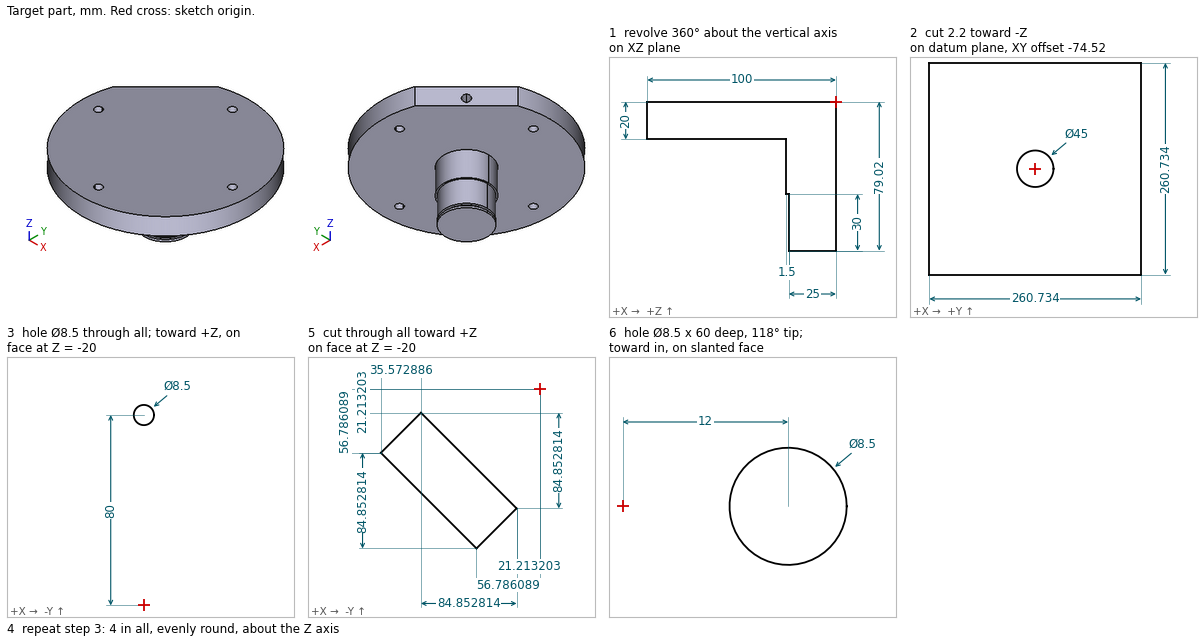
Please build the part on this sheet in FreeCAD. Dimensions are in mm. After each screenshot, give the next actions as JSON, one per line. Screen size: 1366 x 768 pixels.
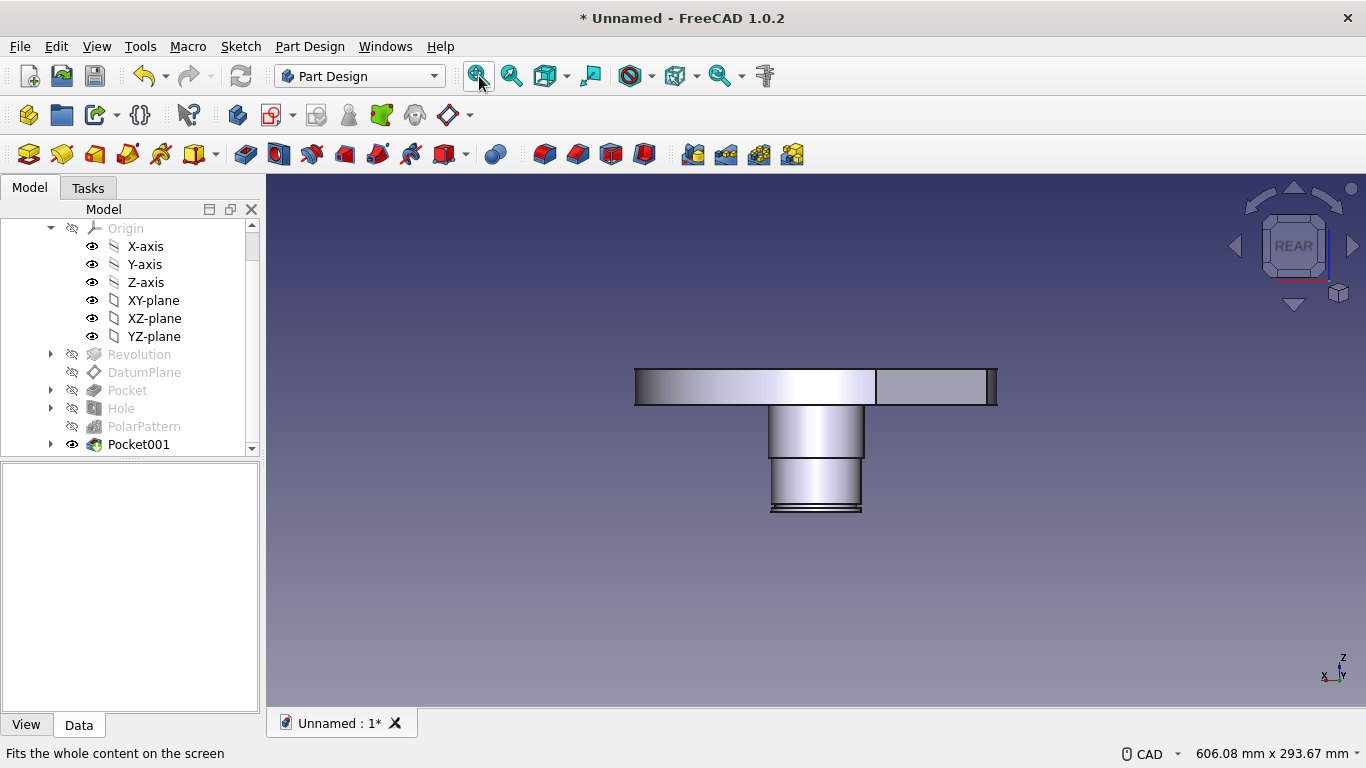
{"action": "left_click", "coordinate": [963, 386]}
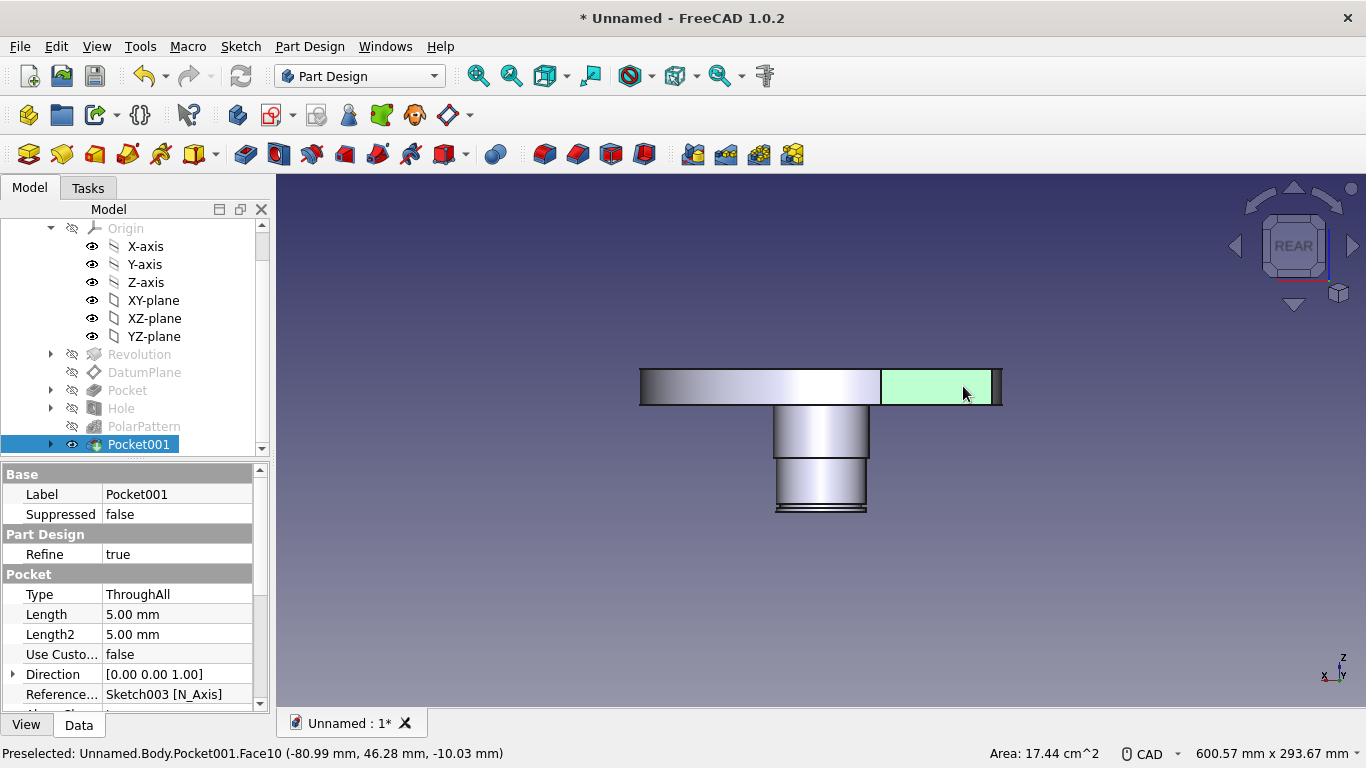
{"action": "left_click", "coordinate": [270, 116]}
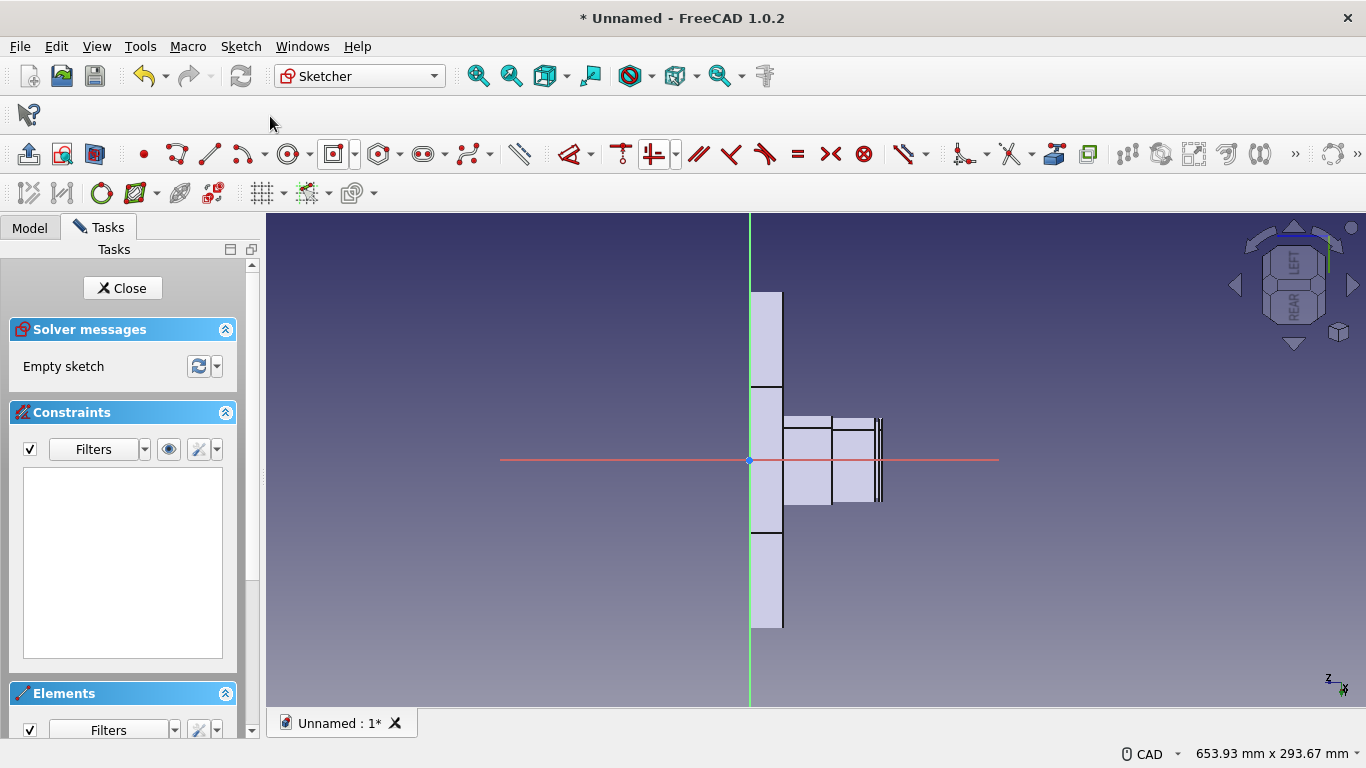
{"action": "left_click", "coordinate": [95, 154]}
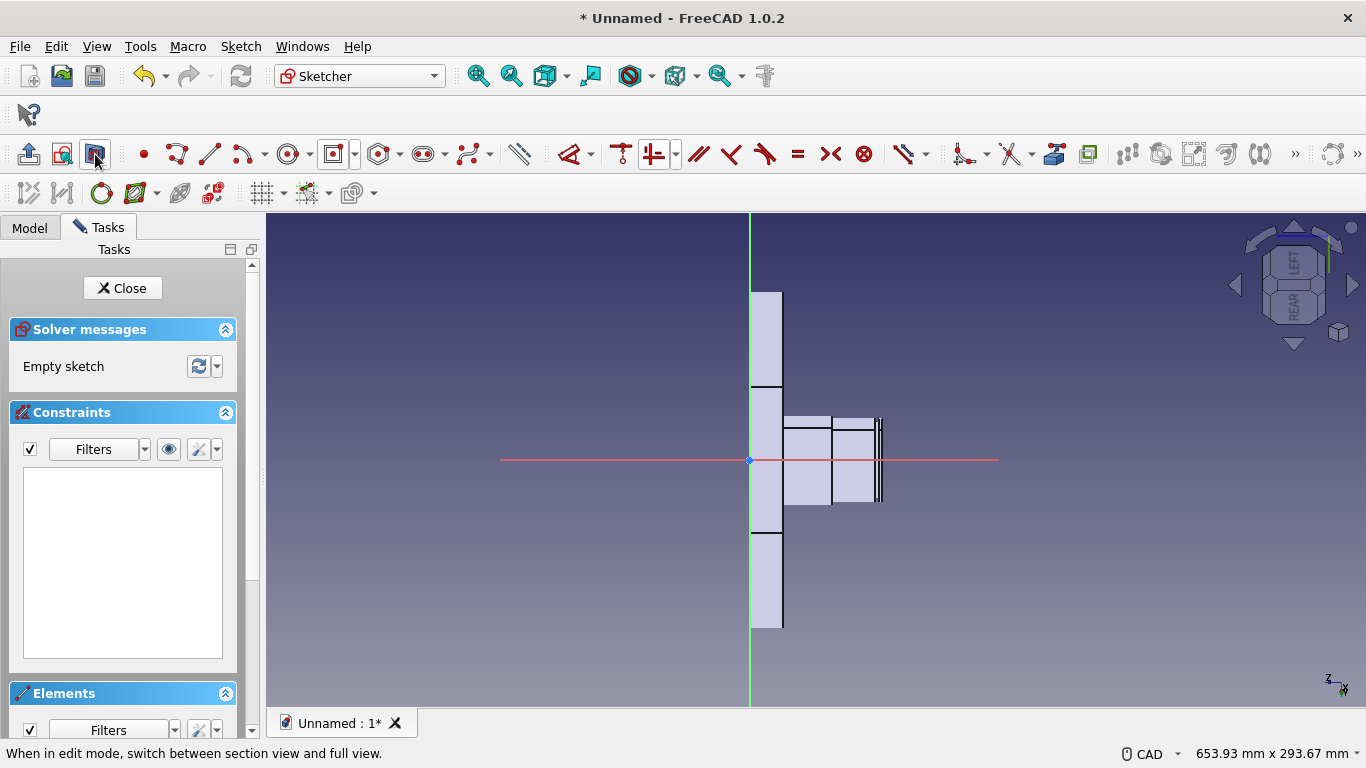
{"action": "scroll", "coordinate": [764, 460], "scroll_direction": "up", "scroll_amount": 15}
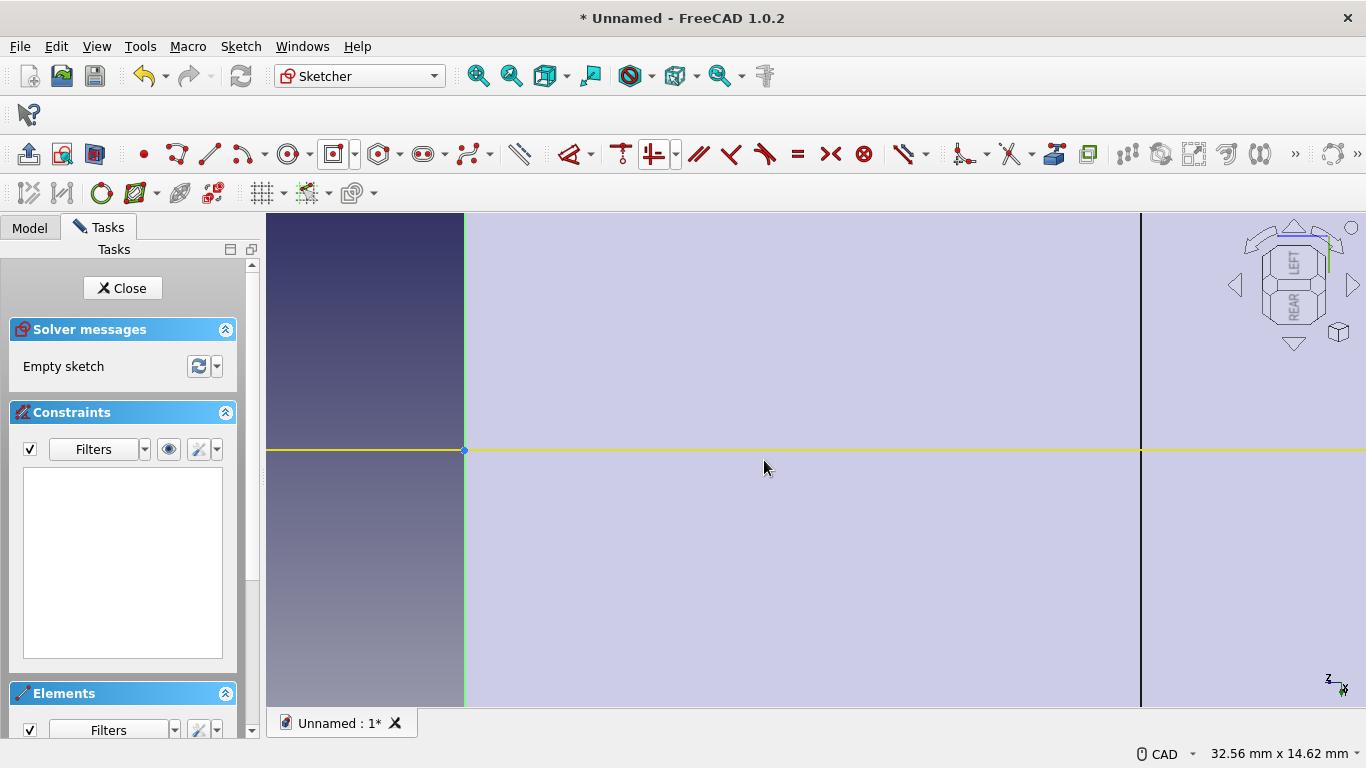
{"action": "left_click", "coordinate": [288, 154]}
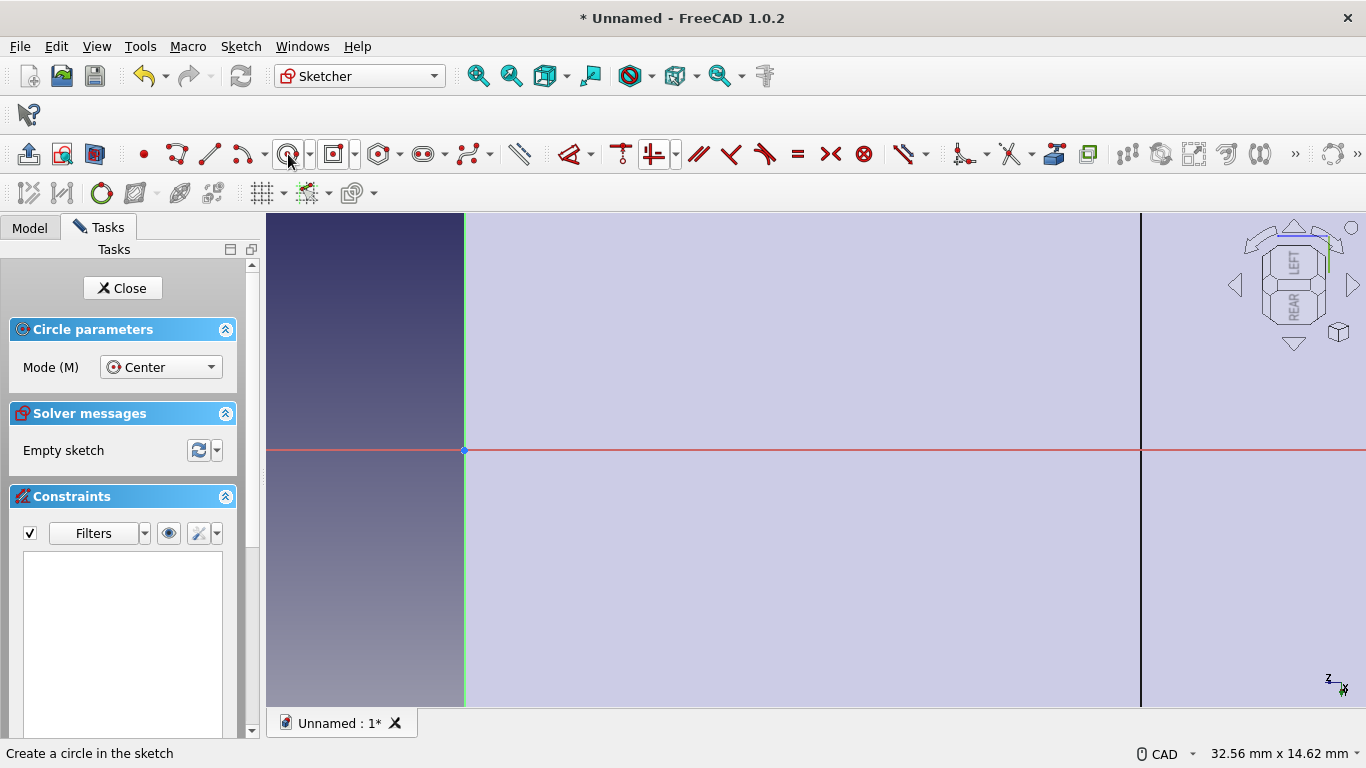
{"action": "left_click", "coordinate": [870, 450]}
{"action": "mouse_move", "coordinate": [972, 349]}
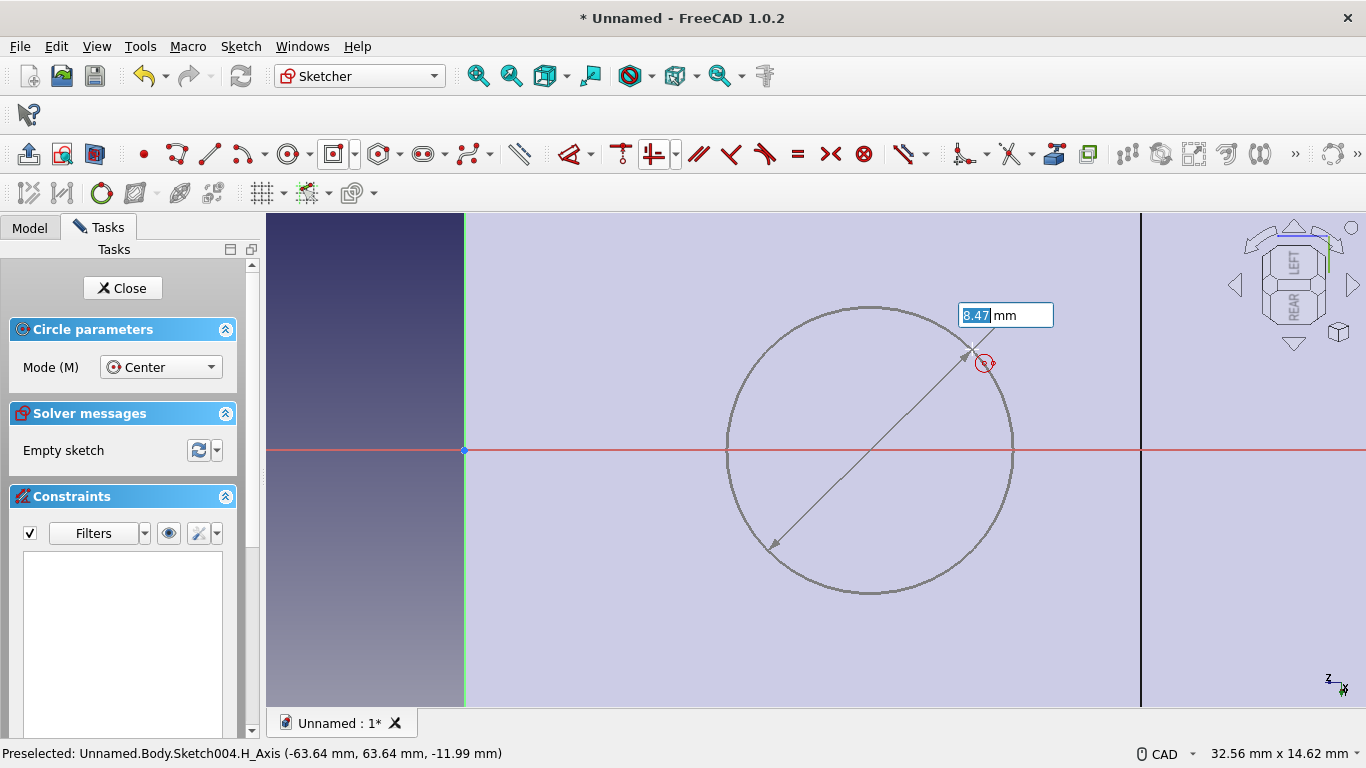
{"action": "type", "text": "8.5"}
{"action": "key", "text": "Return"}
{"action": "key", "text": "Escape"}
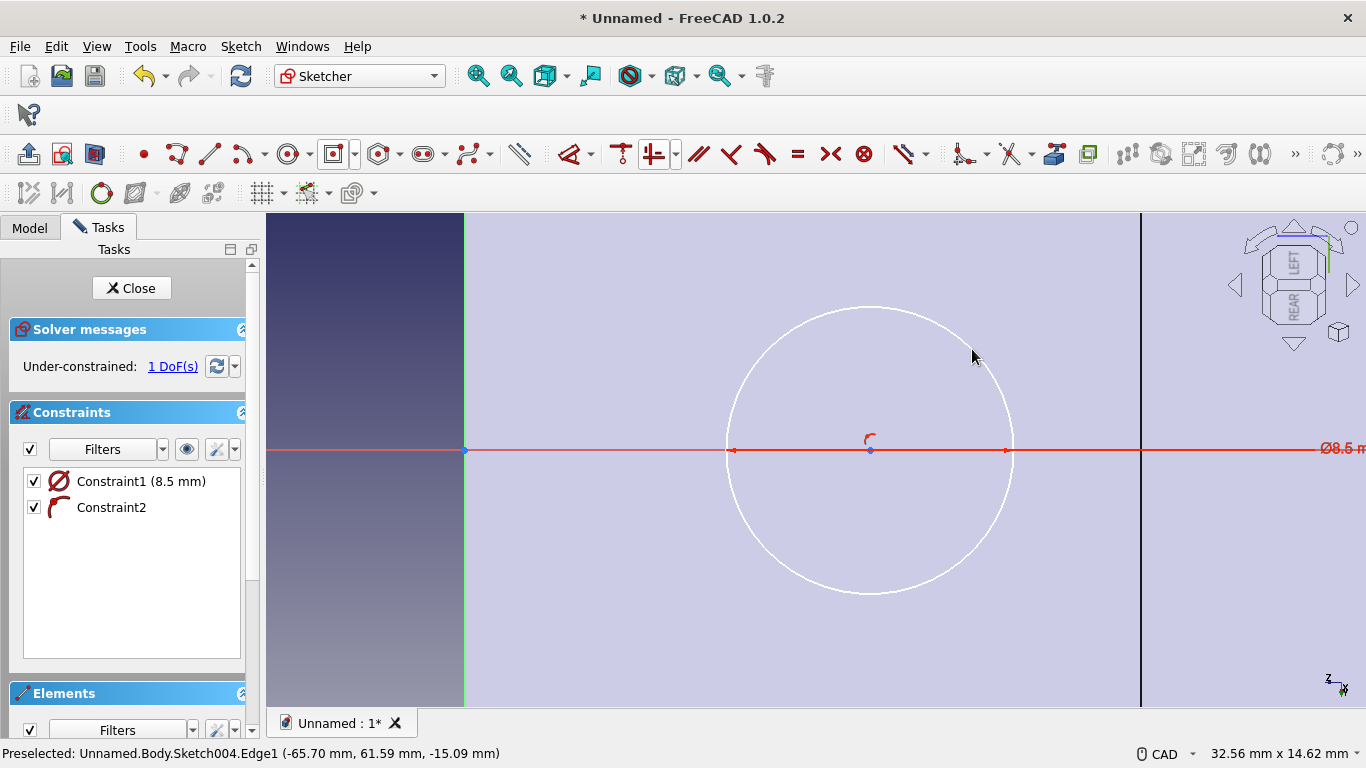
{"action": "left_click", "coordinate": [568, 154]}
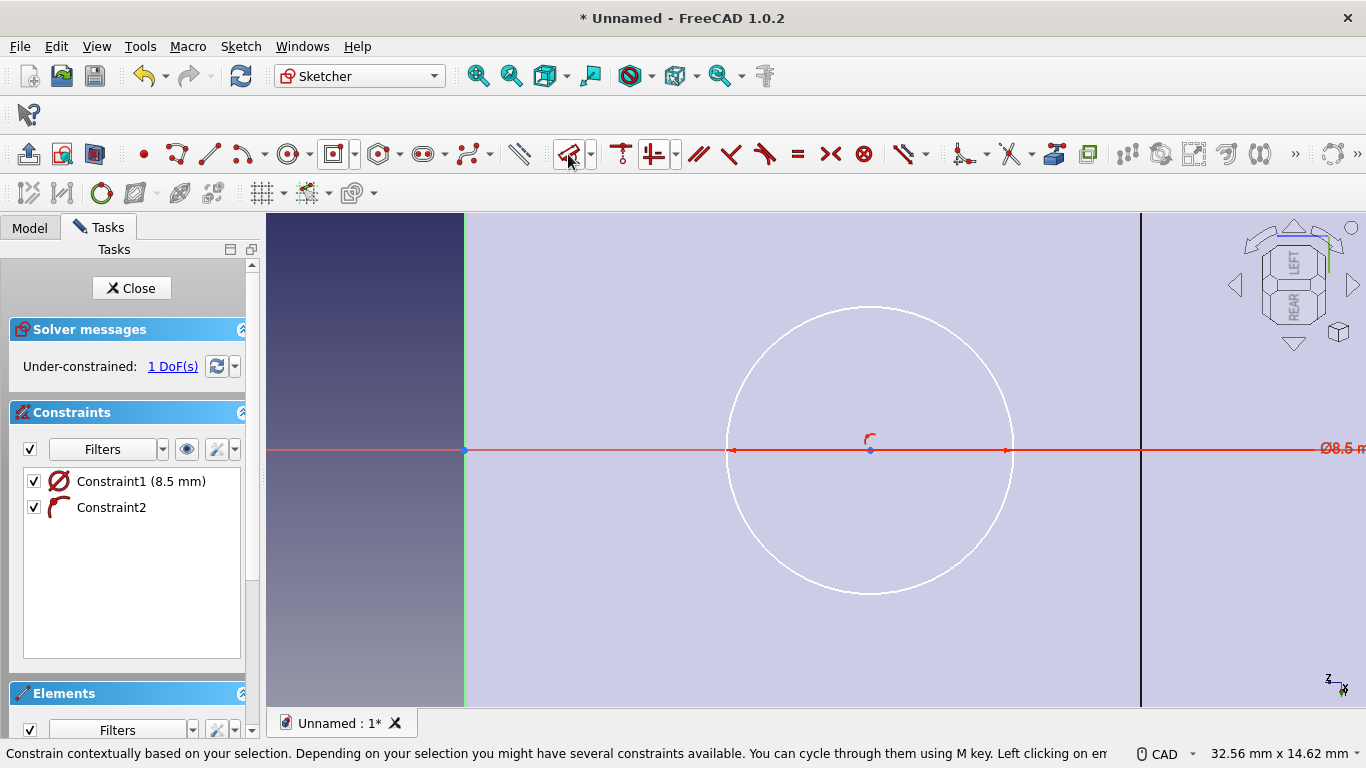
{"action": "left_click", "coordinate": [870, 450]}
{"action": "left_click", "coordinate": [667, 484]}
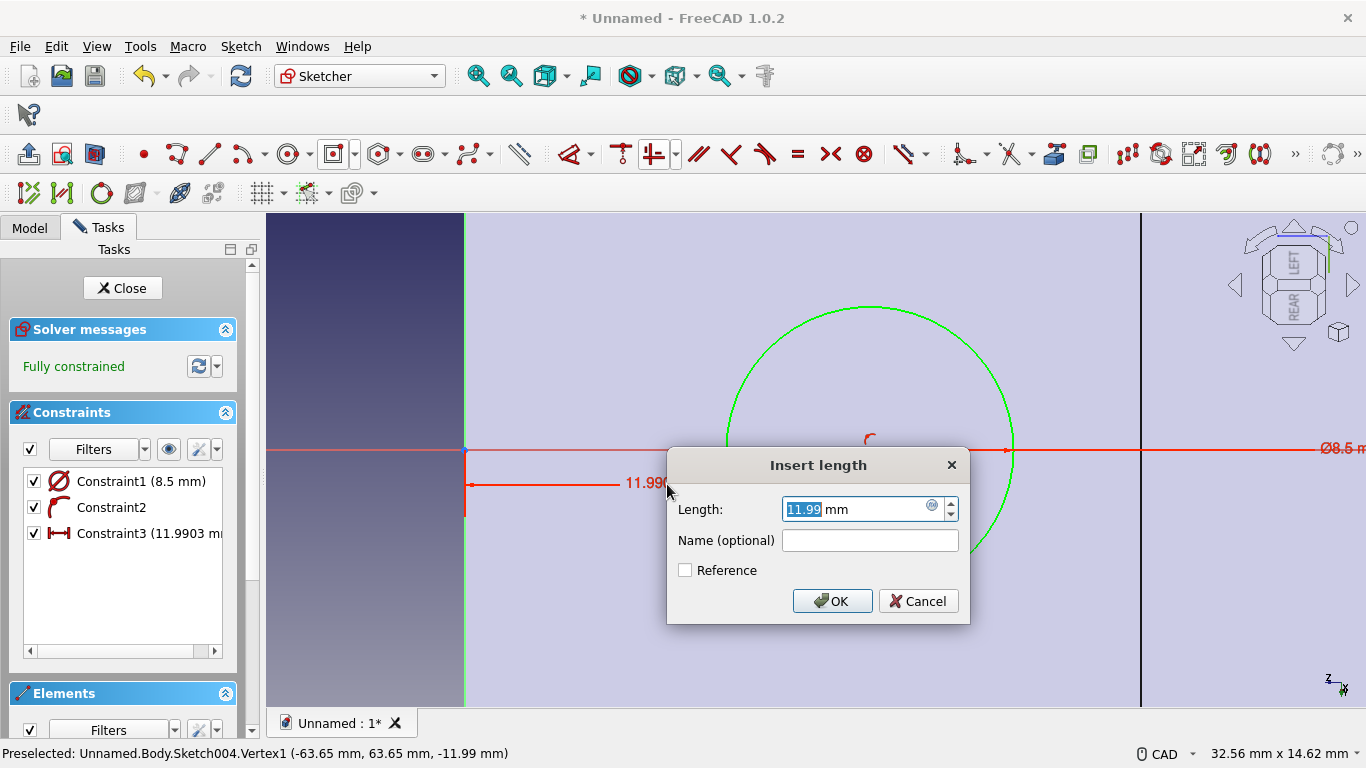
{"action": "type", "text": "12"}
{"action": "key", "text": "Return"}
{"action": "key", "text": "Escape"}